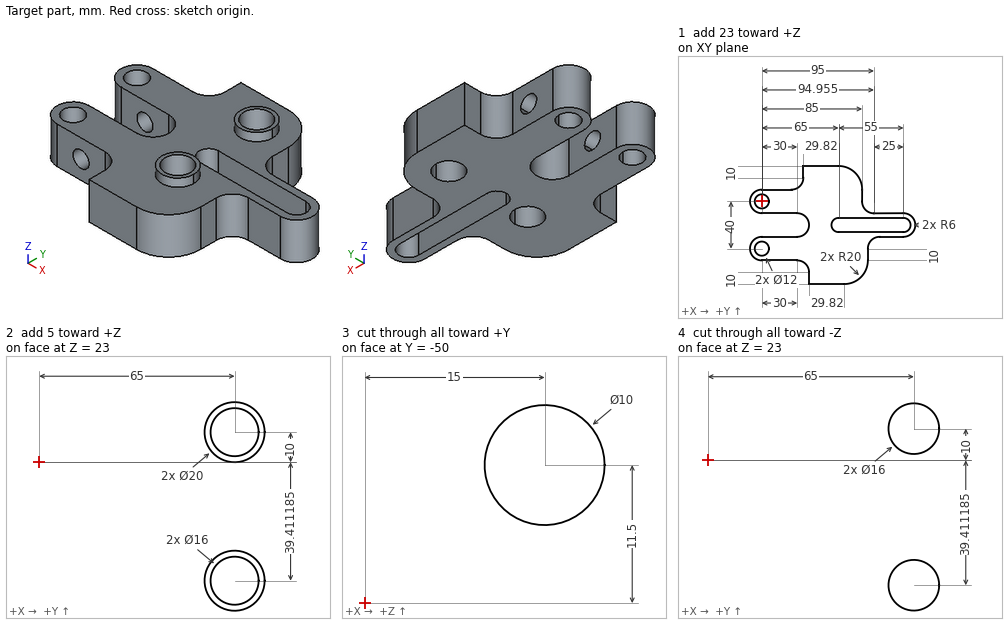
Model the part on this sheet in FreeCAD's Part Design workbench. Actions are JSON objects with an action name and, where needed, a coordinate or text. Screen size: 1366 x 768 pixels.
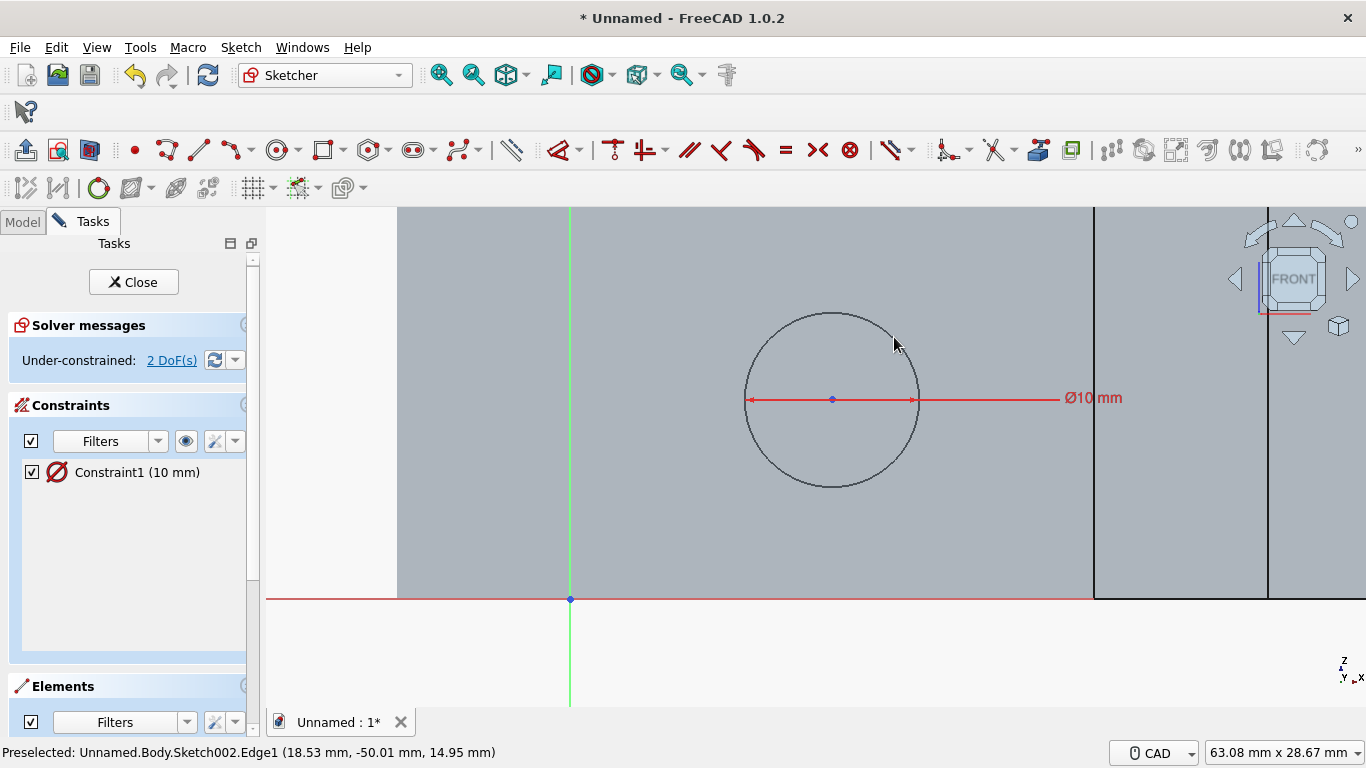
{"action": "left_click", "coordinate": [558, 150]}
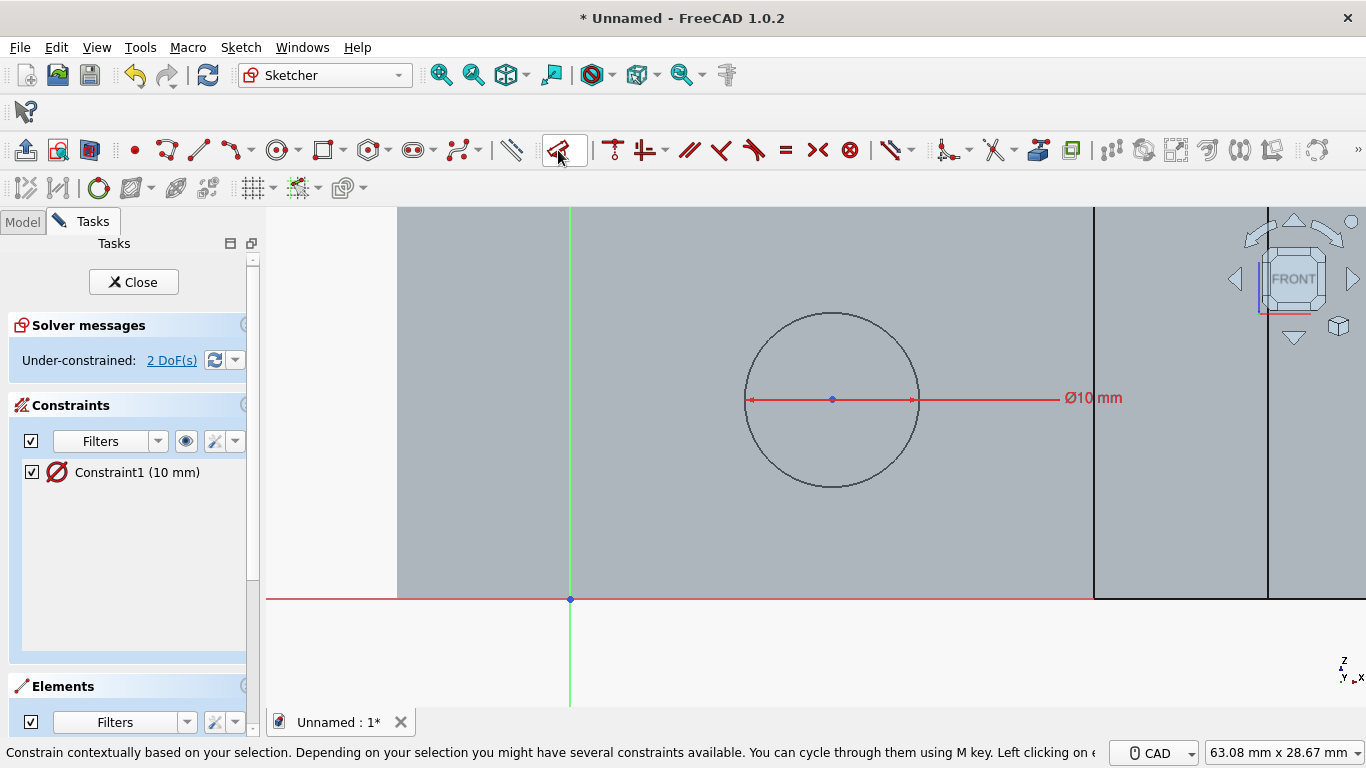
{"action": "left_click", "coordinate": [832, 400]}
{"action": "left_click", "coordinate": [701, 633]}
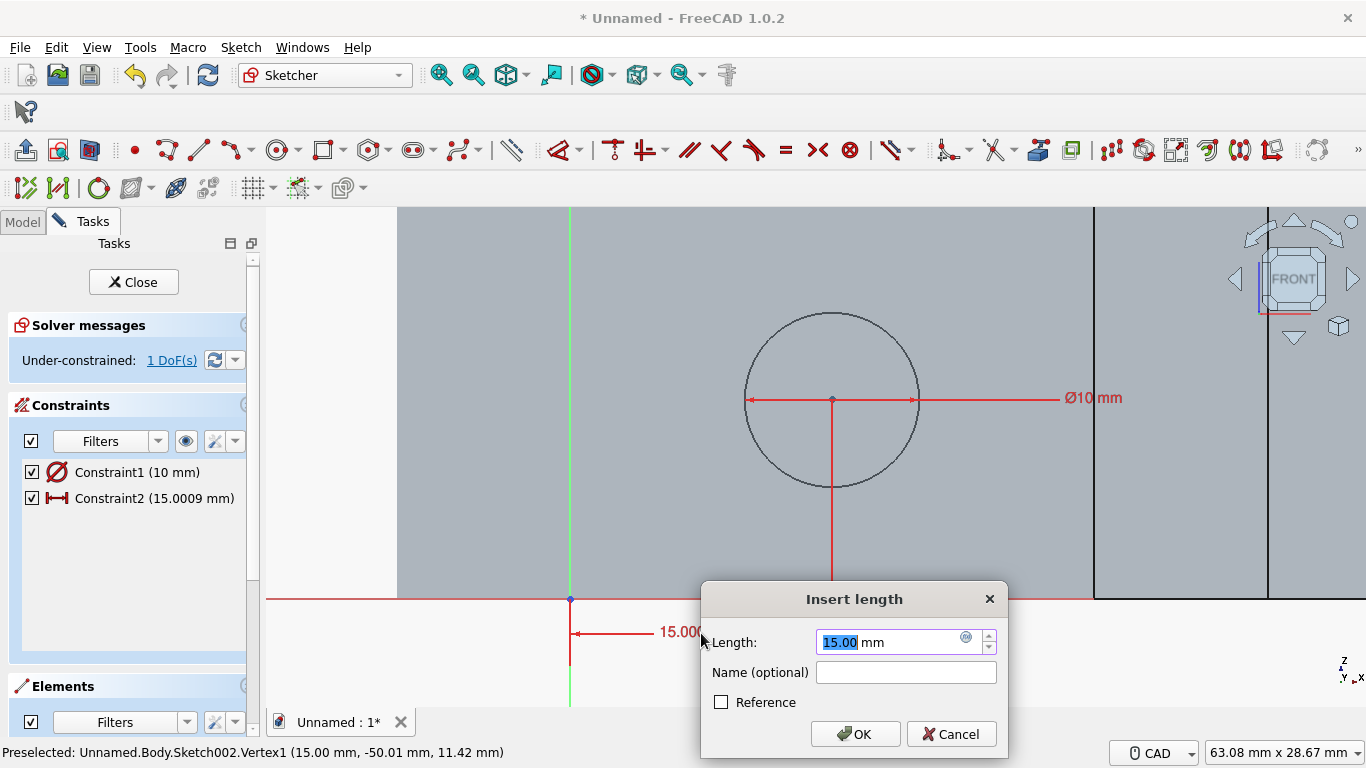
{"action": "type", "text": "15"}
{"action": "key", "text": "Return"}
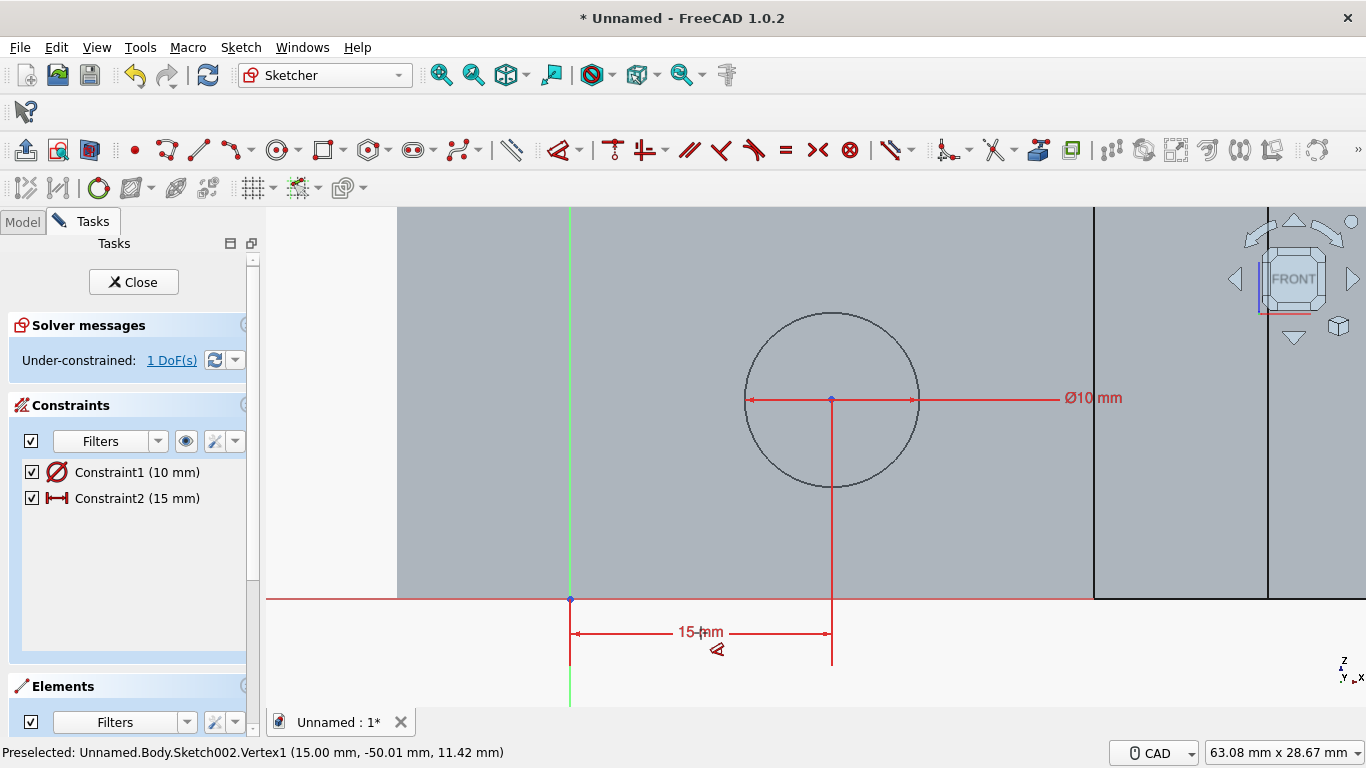
{"action": "left_click", "coordinate": [832, 400]}
{"action": "left_click", "coordinate": [536, 500]}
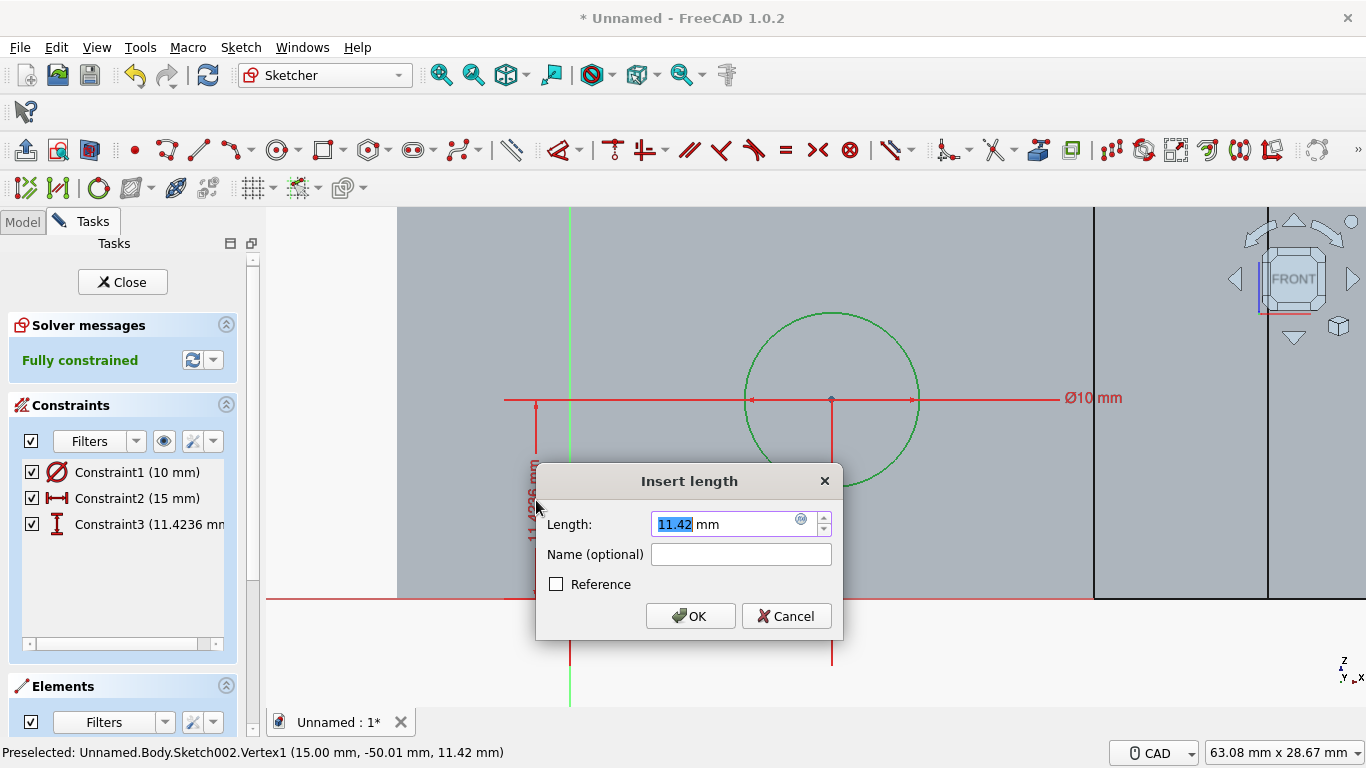
{"action": "type", "text": "11.5"}
{"action": "key", "text": "Return"}
{"action": "key", "text": "Escape"}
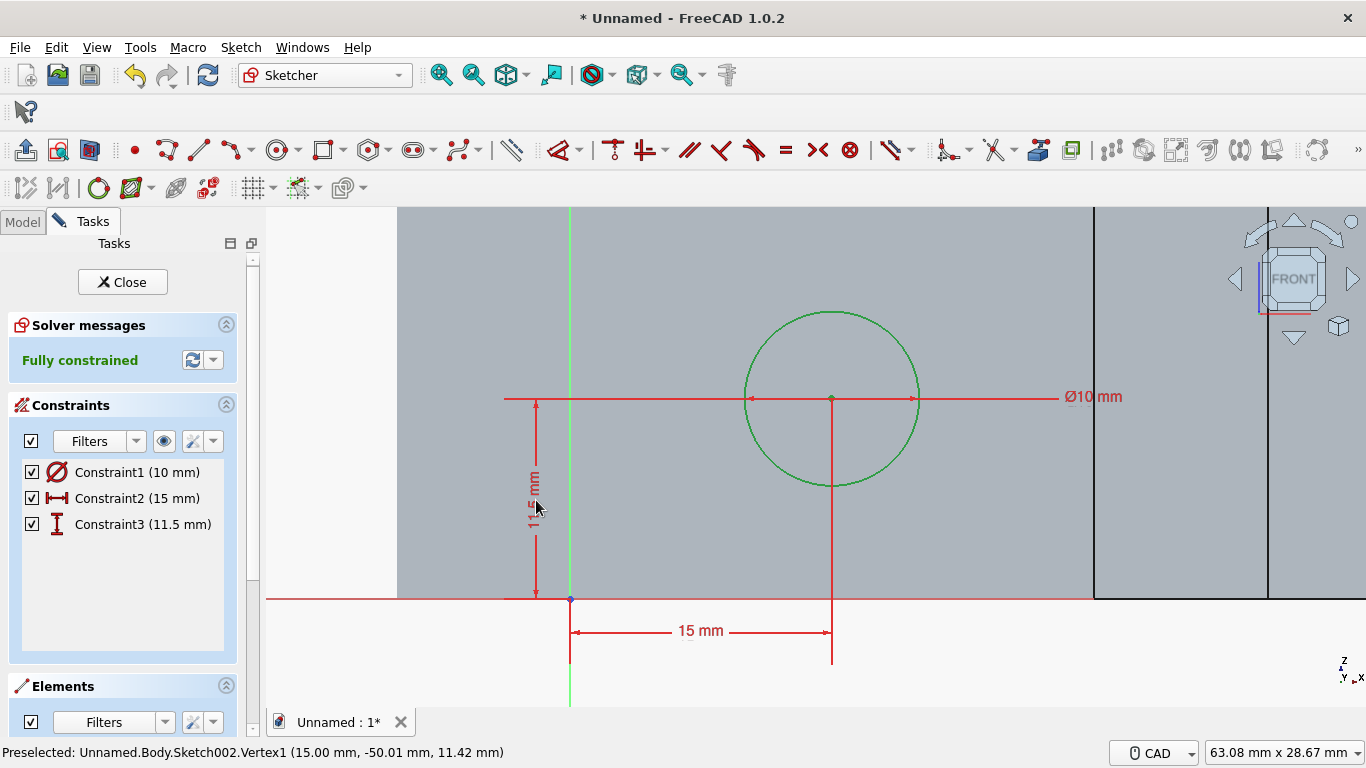
{"action": "left_click", "coordinate": [123, 282]}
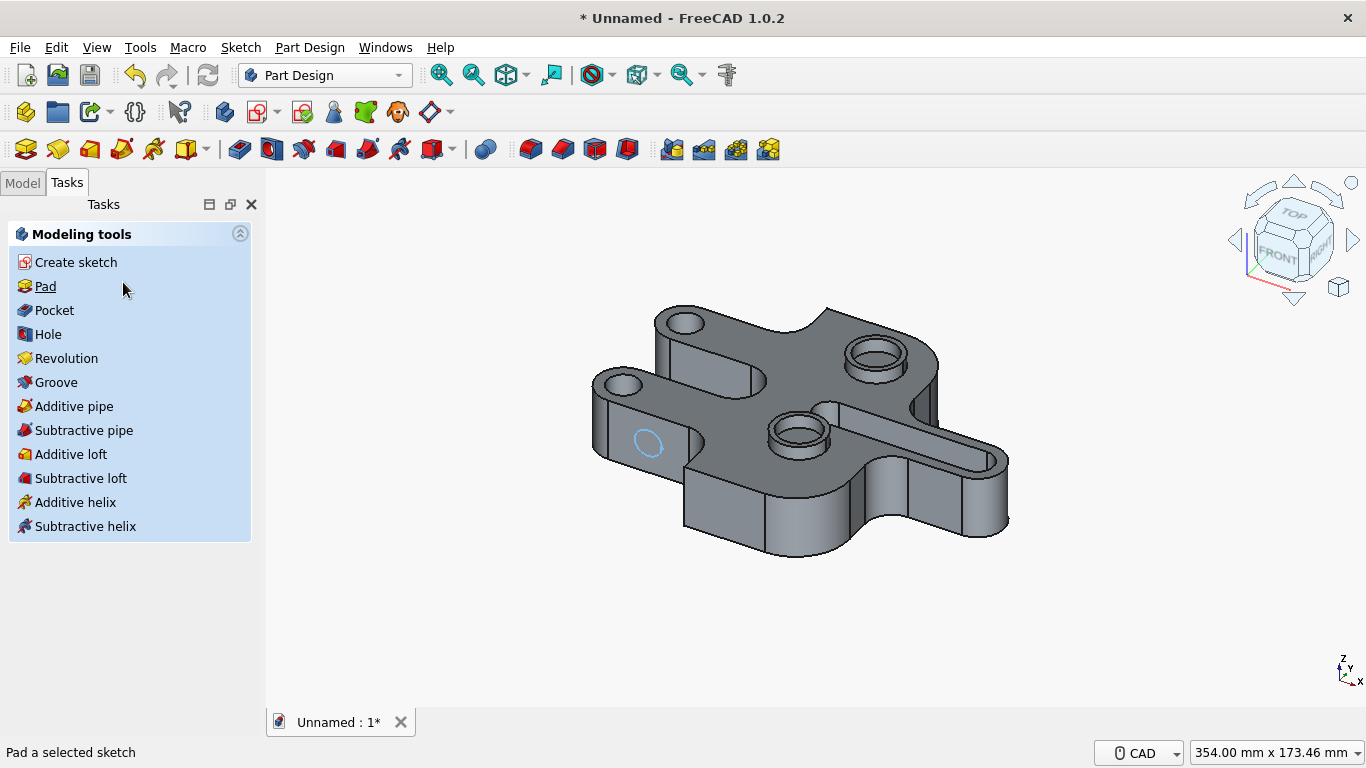
{"action": "left_click", "coordinate": [240, 150]}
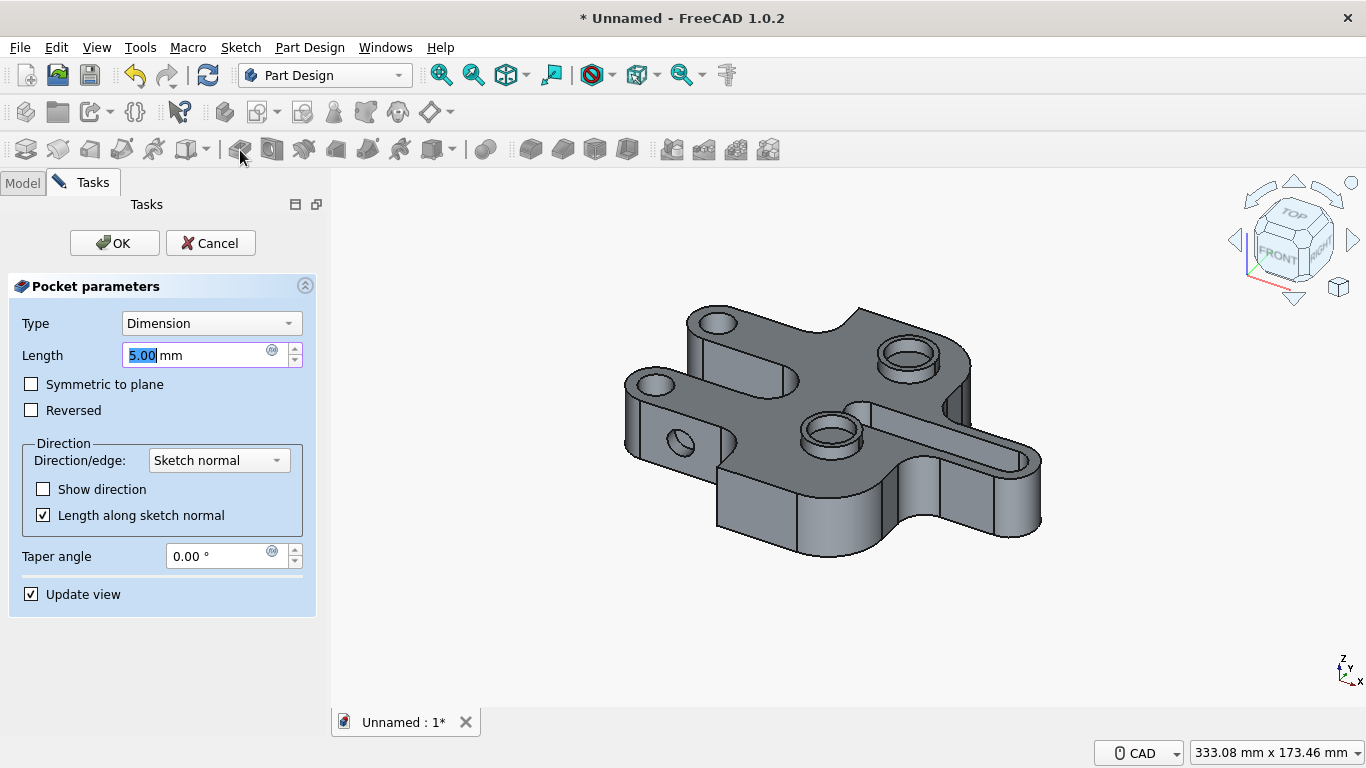
{"action": "left_click", "coordinate": [212, 324]}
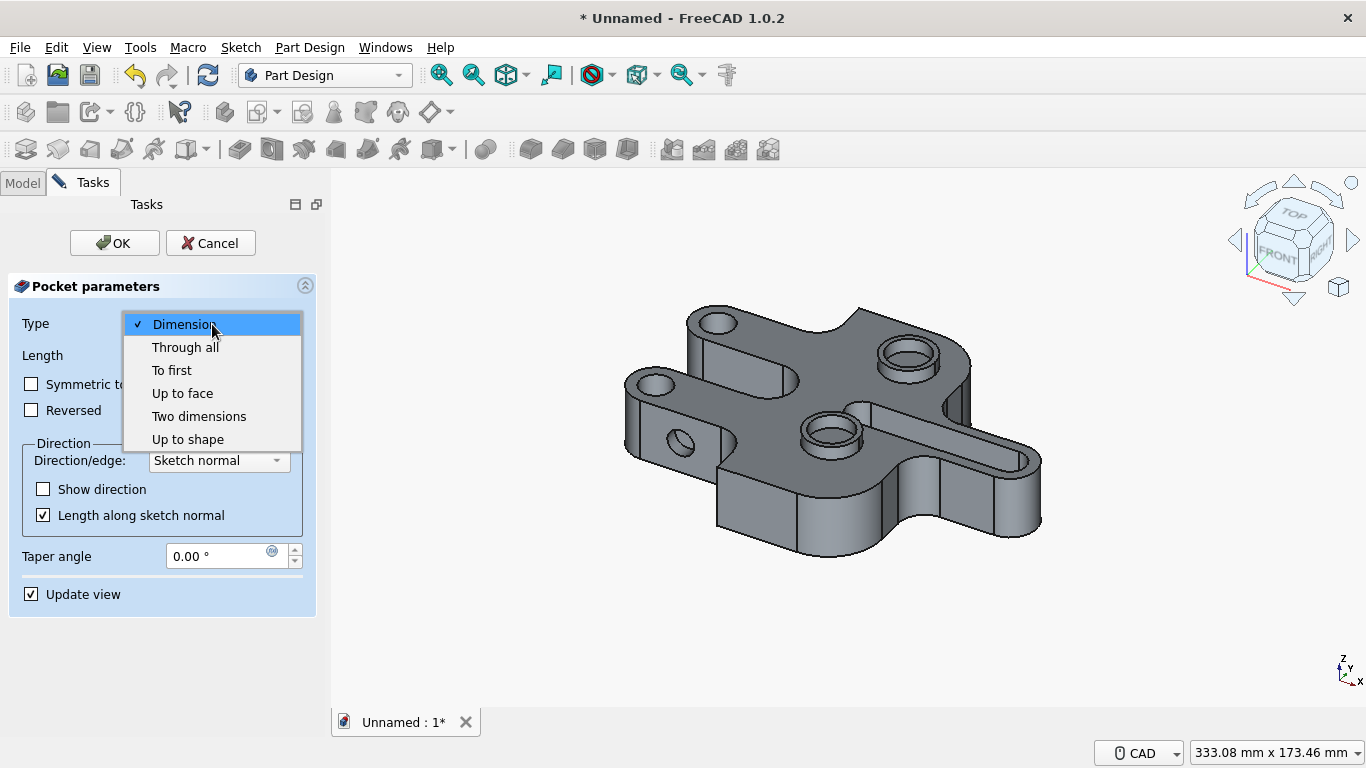
{"action": "left_click", "coordinate": [212, 348]}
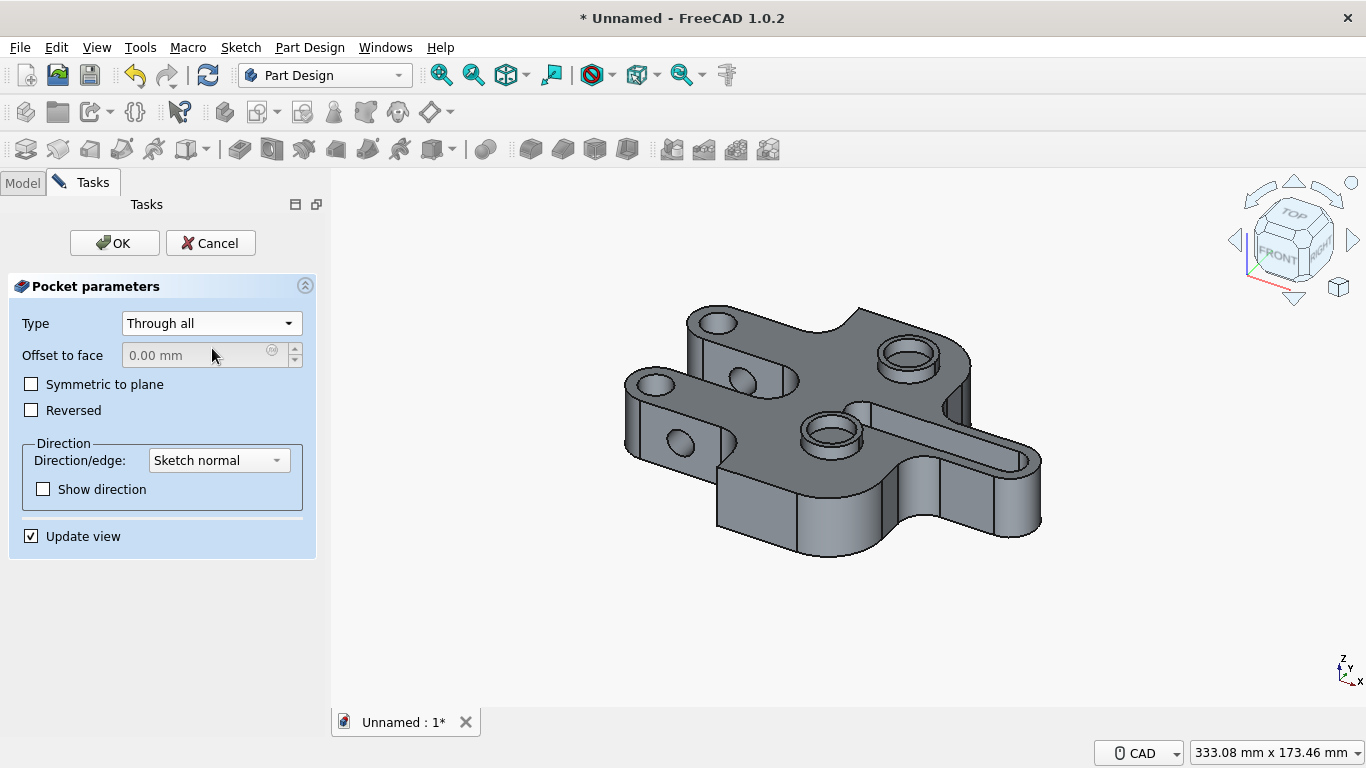
{"action": "left_click", "coordinate": [115, 243]}